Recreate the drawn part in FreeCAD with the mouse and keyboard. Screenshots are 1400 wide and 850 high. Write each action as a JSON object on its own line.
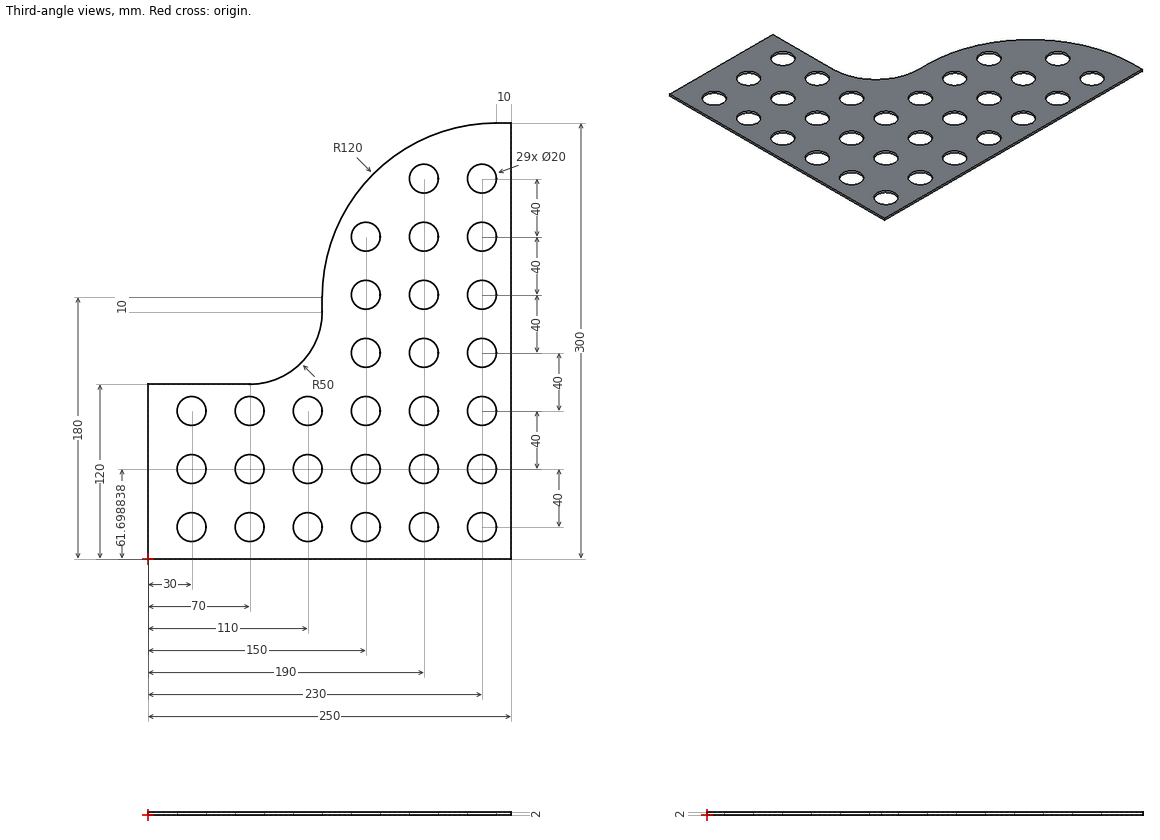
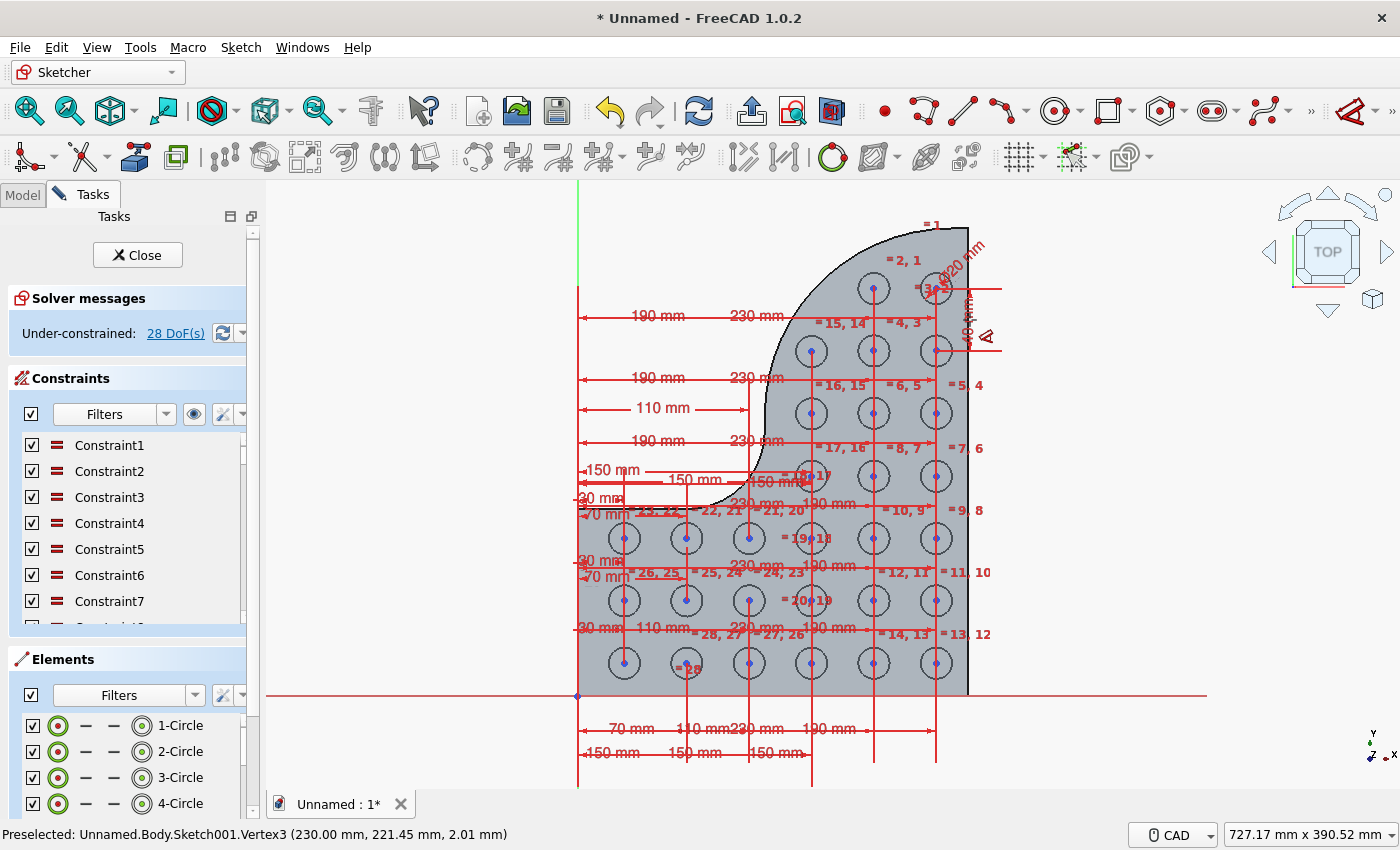
{"action": "left_click", "coordinate": [874, 289]}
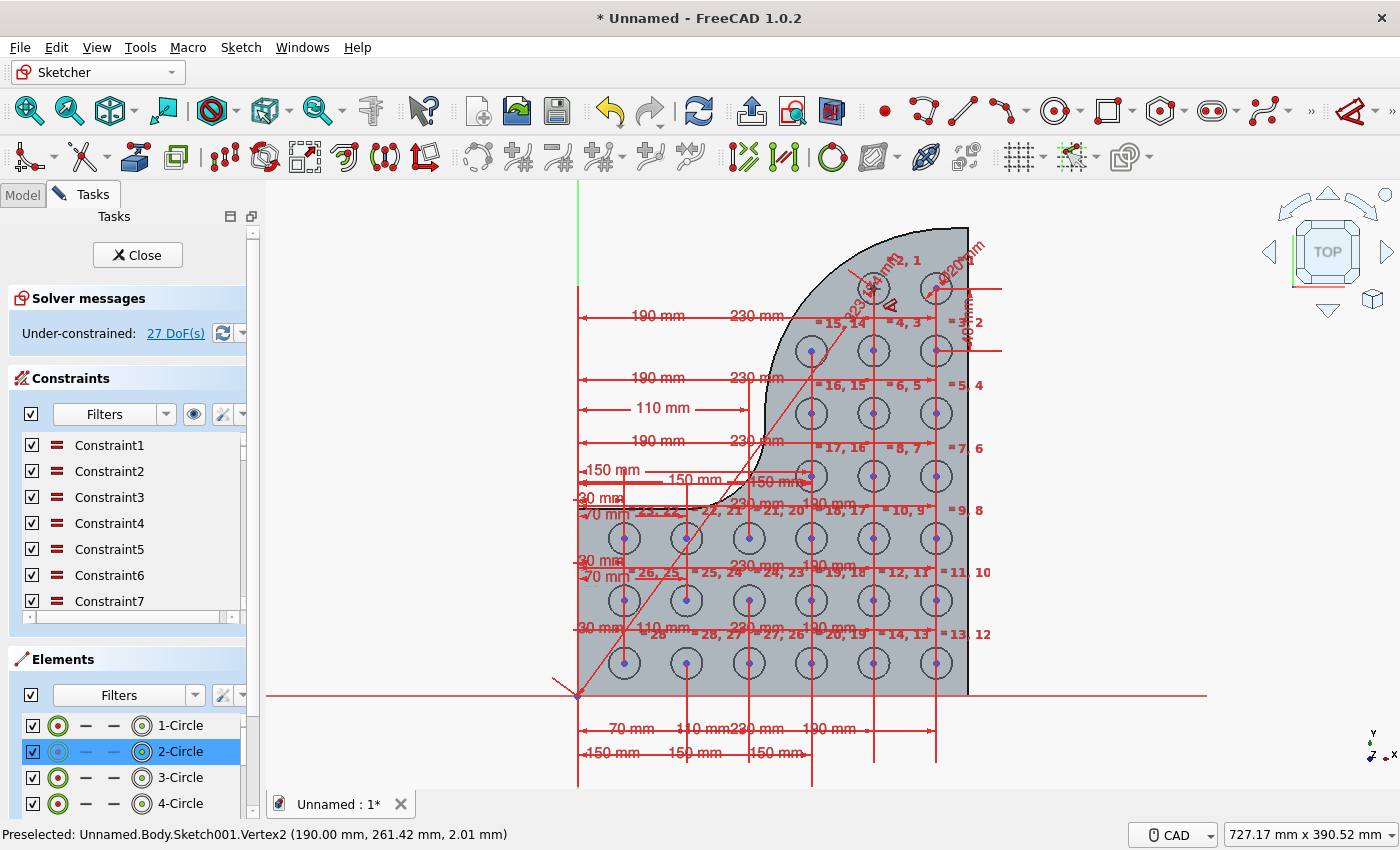
{"action": "left_click", "coordinate": [936, 351]}
{"action": "left_click", "coordinate": [970, 298]}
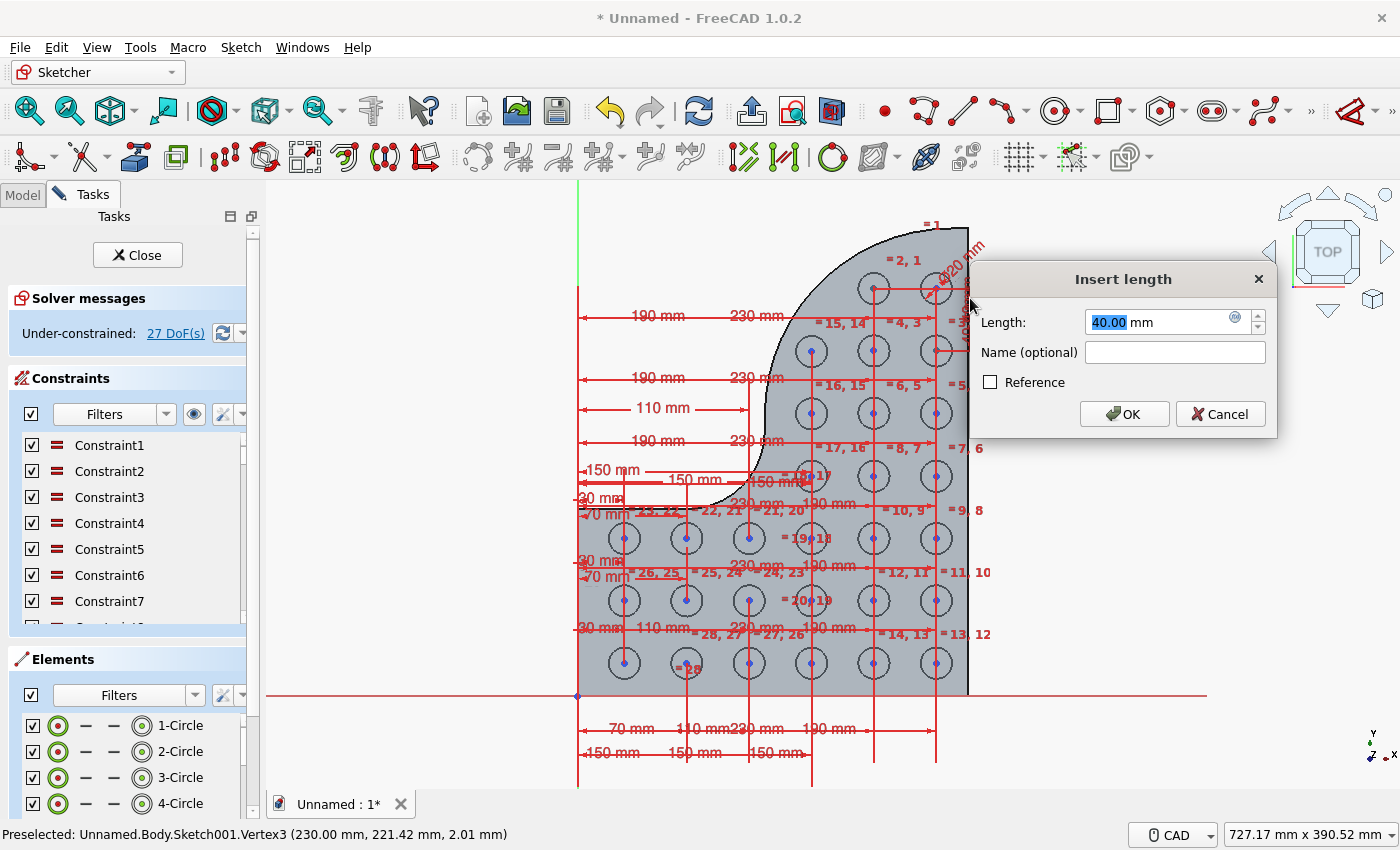
{"action": "type", "text": "40"}
{"action": "key", "text": "Return"}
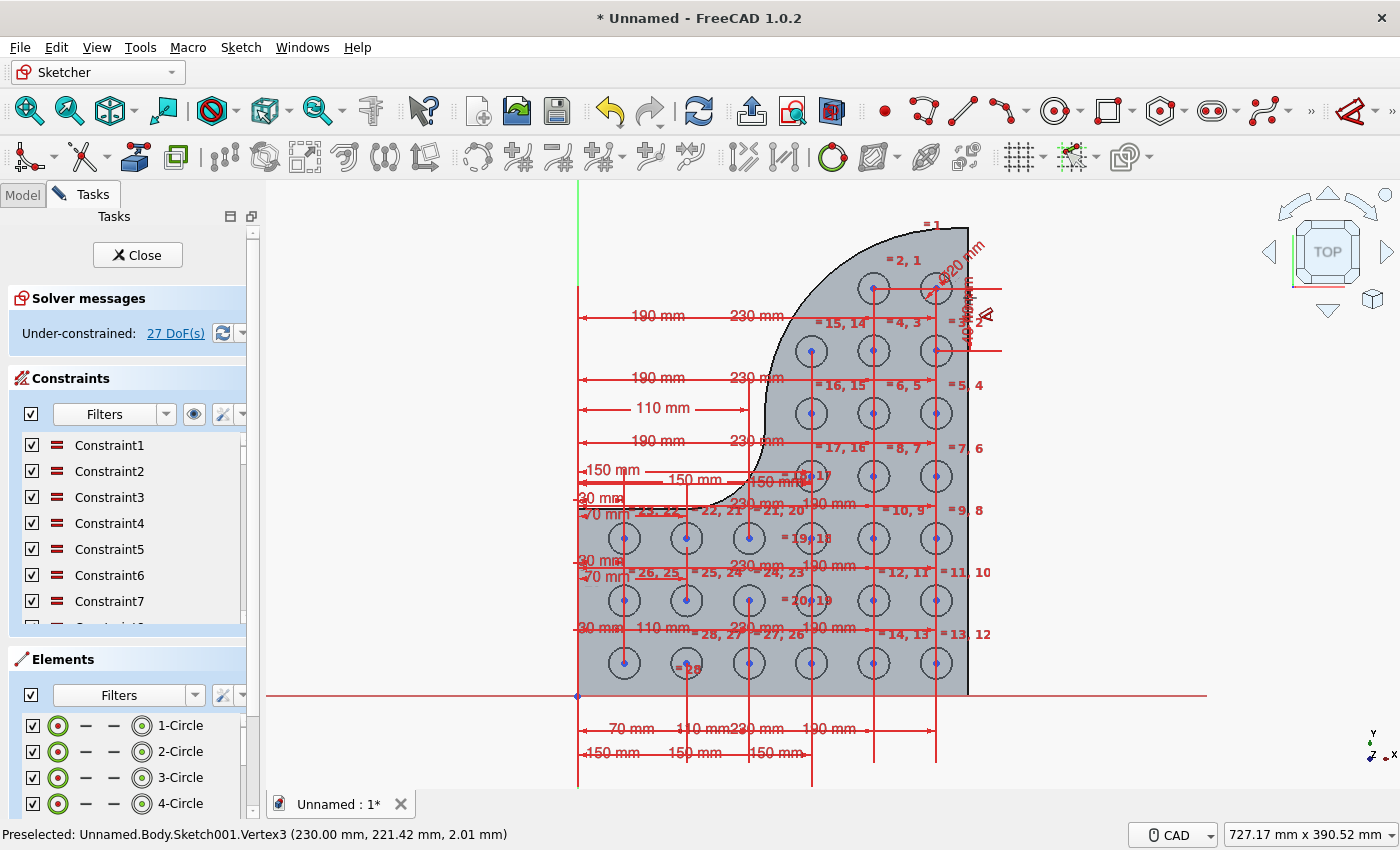
{"action": "left_click", "coordinate": [874, 289]}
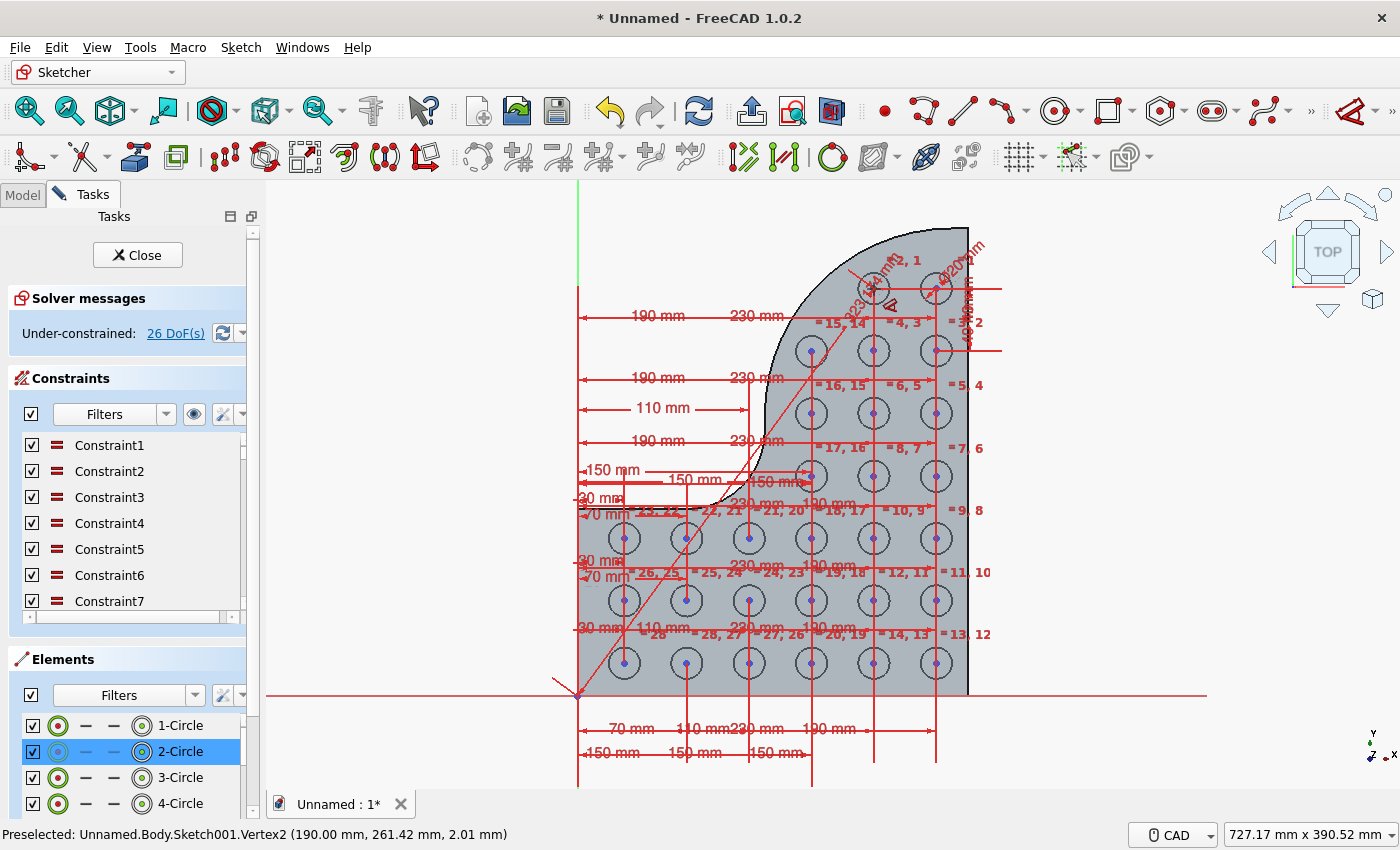
{"action": "left_click", "coordinate": [874, 351]}
{"action": "left_click", "coordinate": [908, 342]}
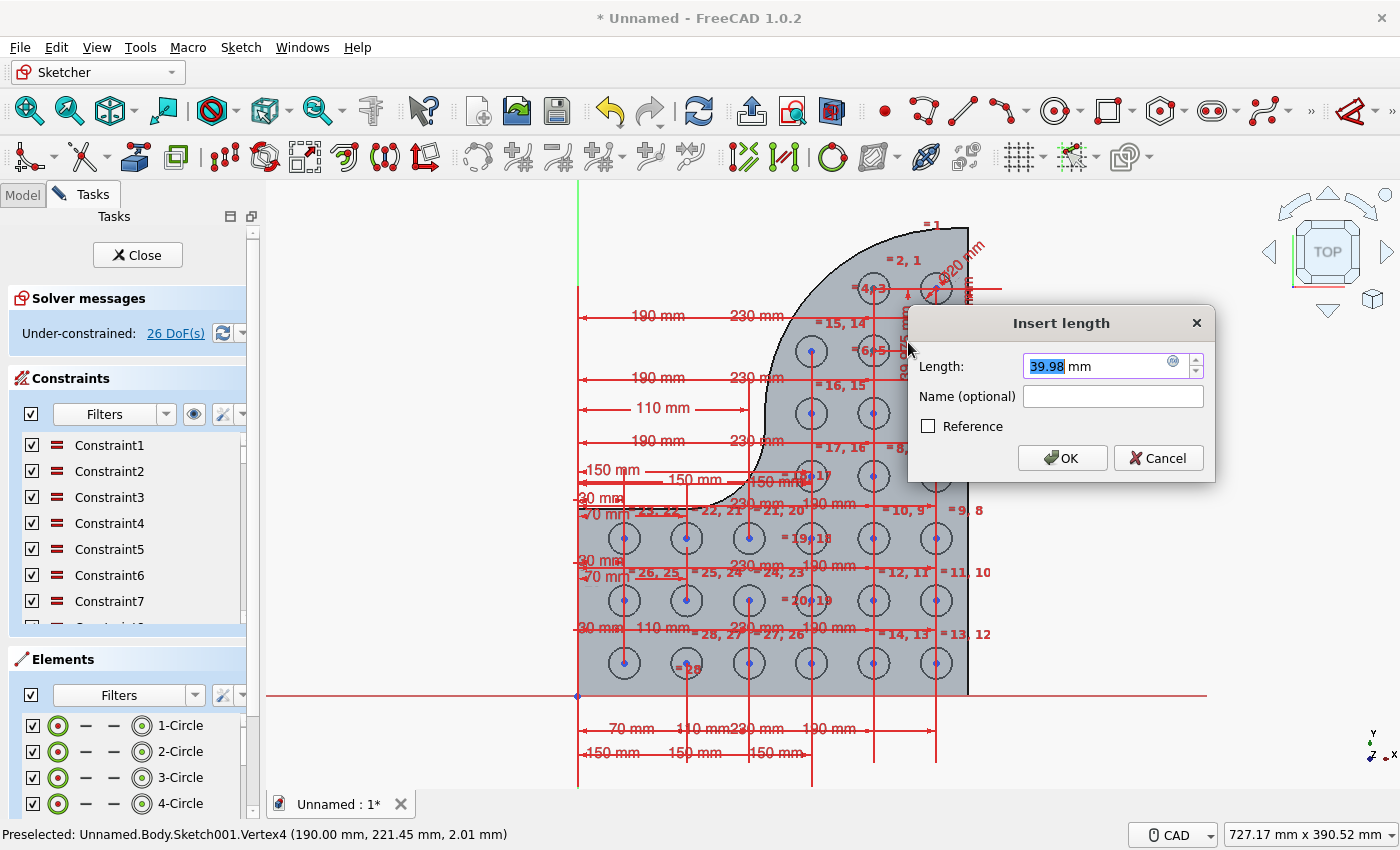
{"action": "type", "text": "40"}
{"action": "key", "text": "Return"}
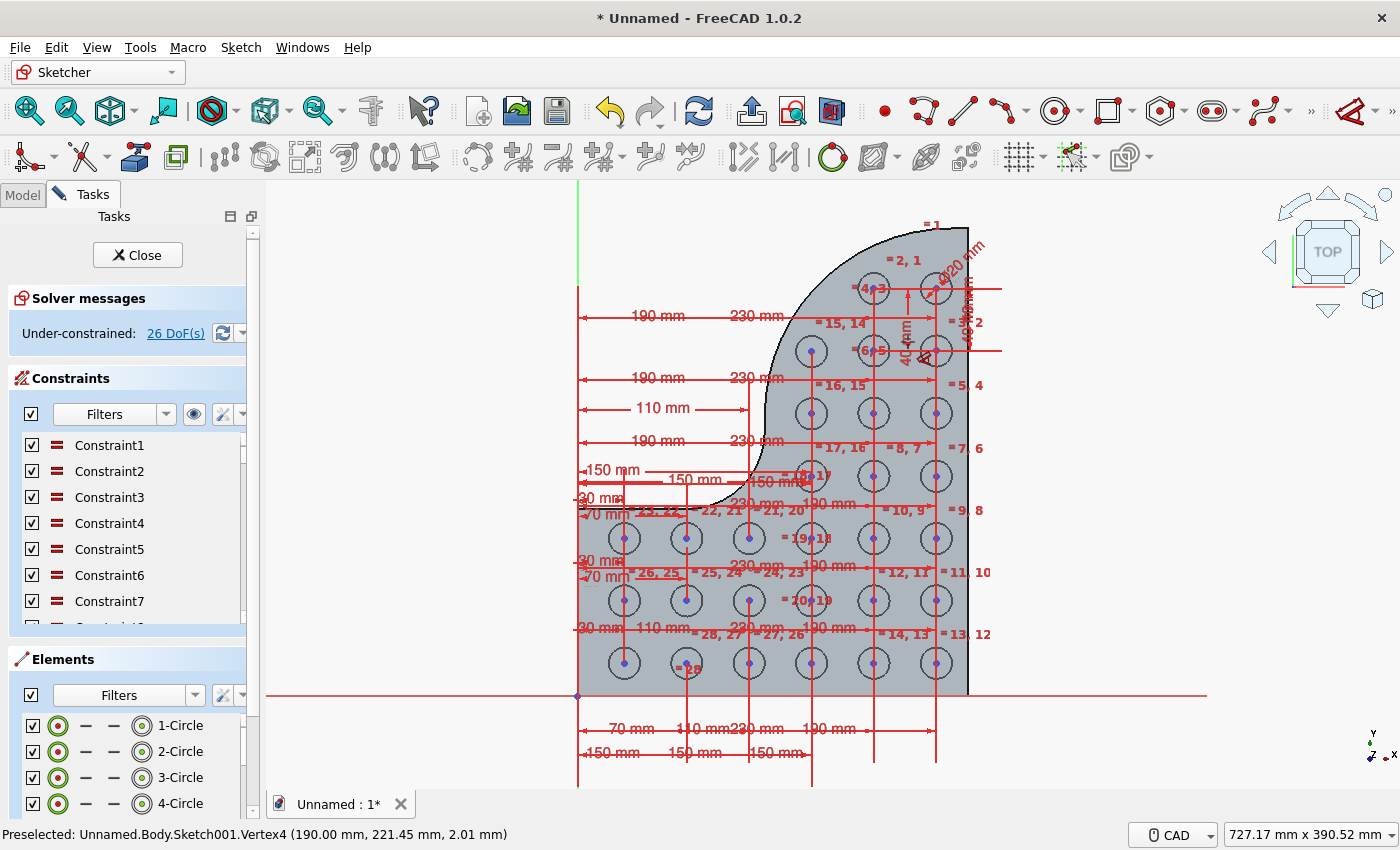
{"action": "left_click", "coordinate": [936, 351]}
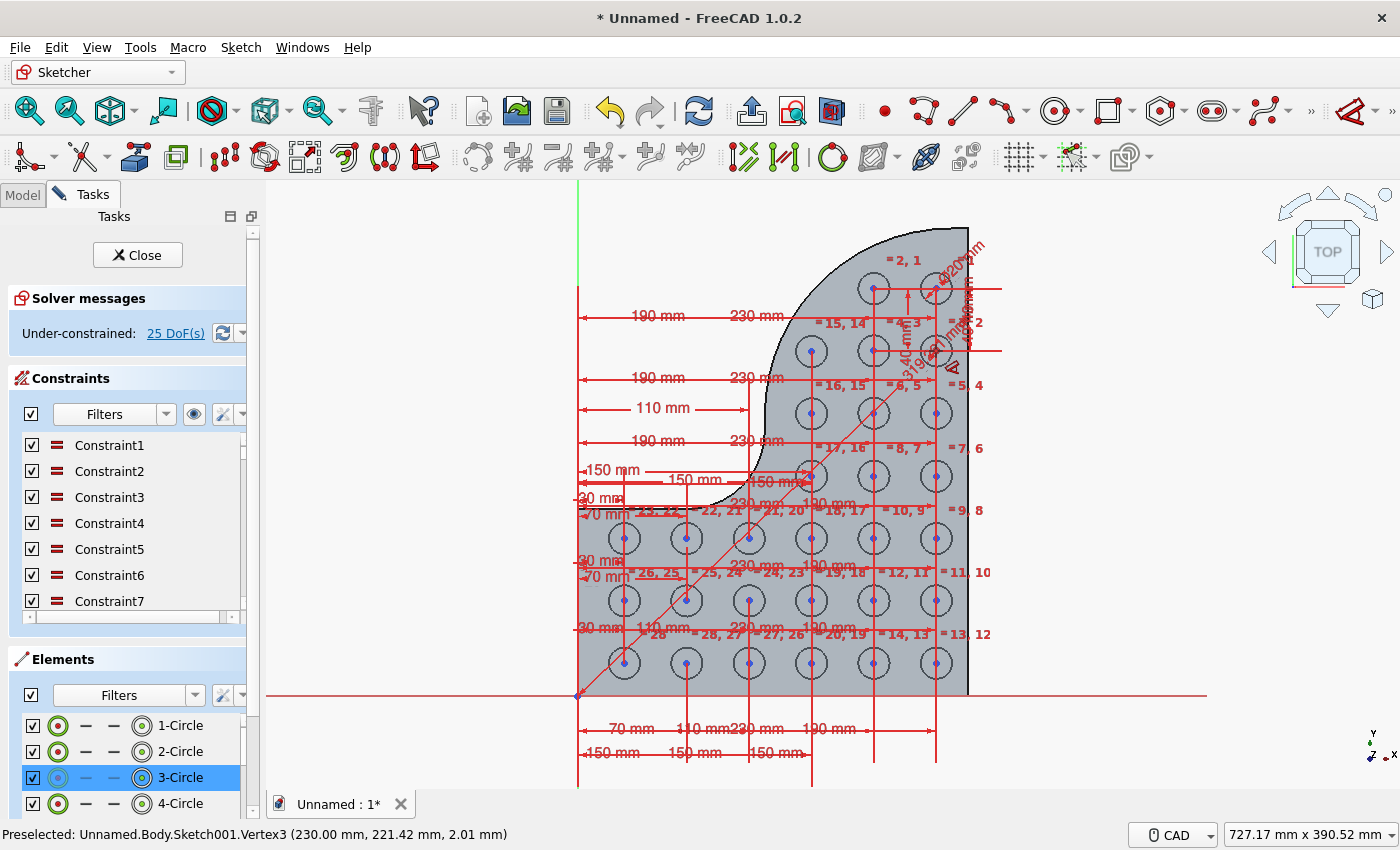
{"action": "left_click", "coordinate": [936, 413]}
{"action": "left_click", "coordinate": [970, 382]}